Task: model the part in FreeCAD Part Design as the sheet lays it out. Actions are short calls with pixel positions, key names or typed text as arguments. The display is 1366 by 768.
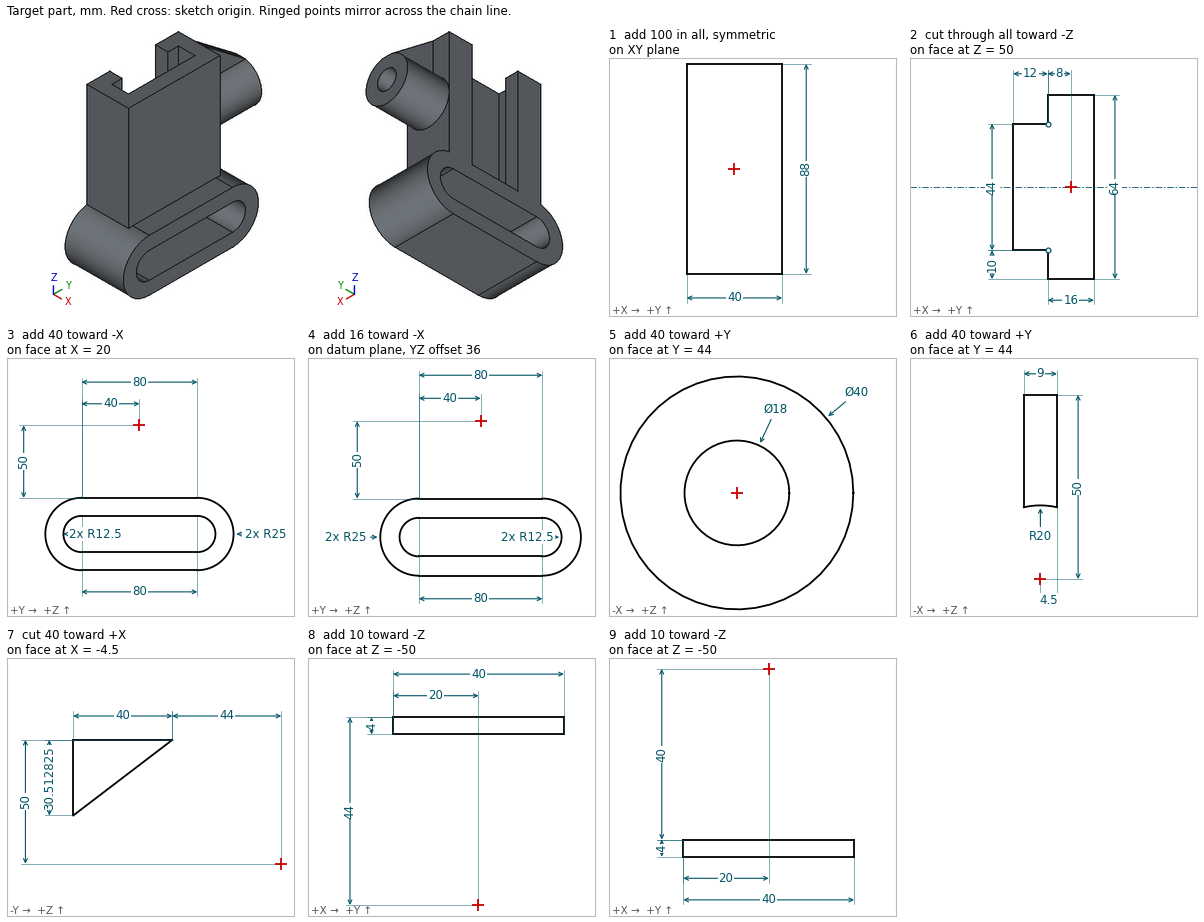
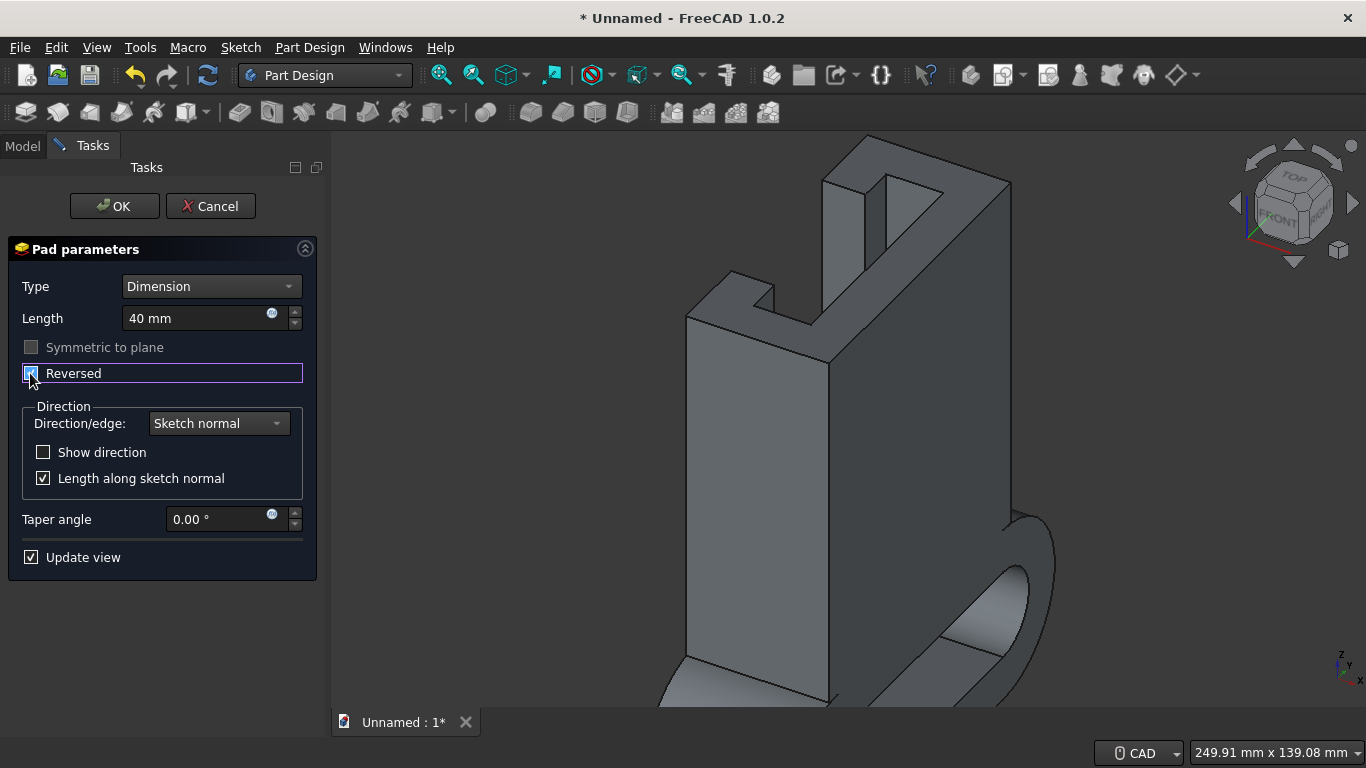
click(115, 206)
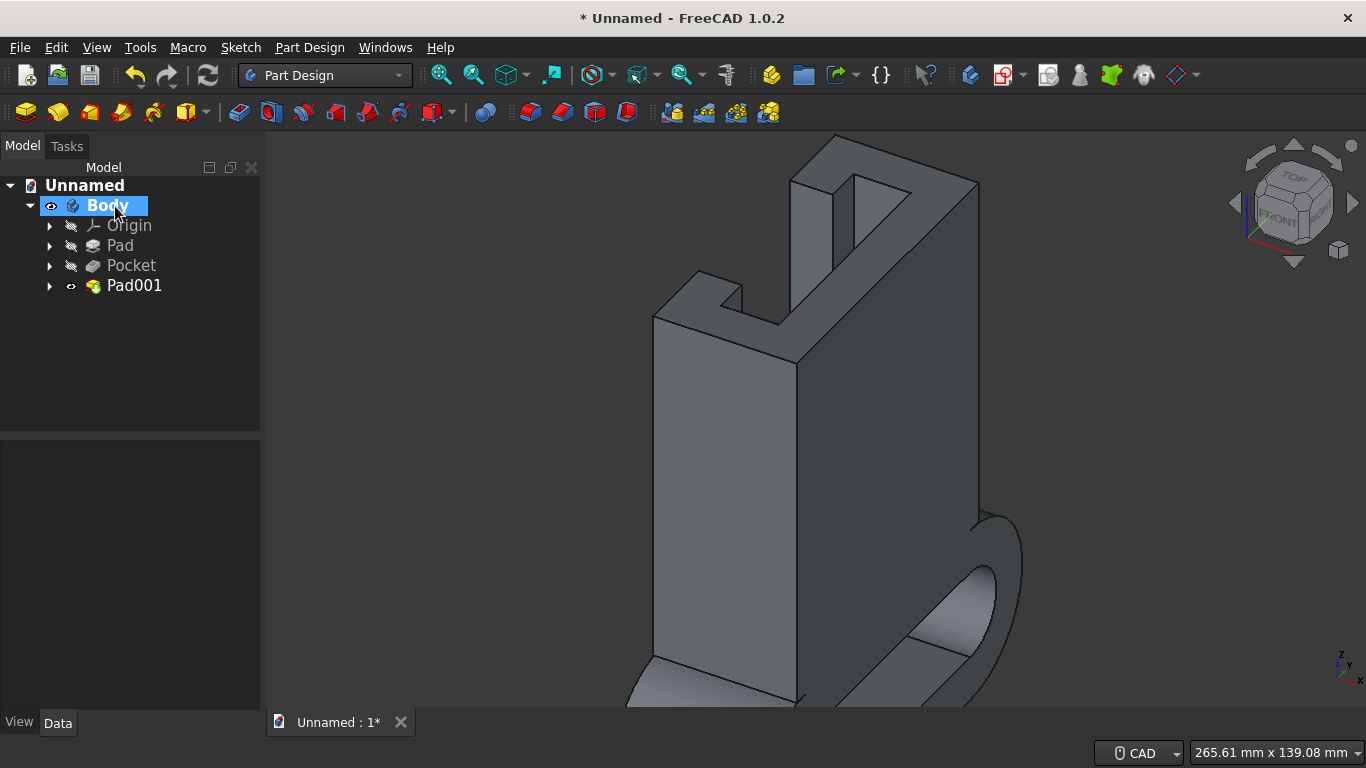
click(442, 76)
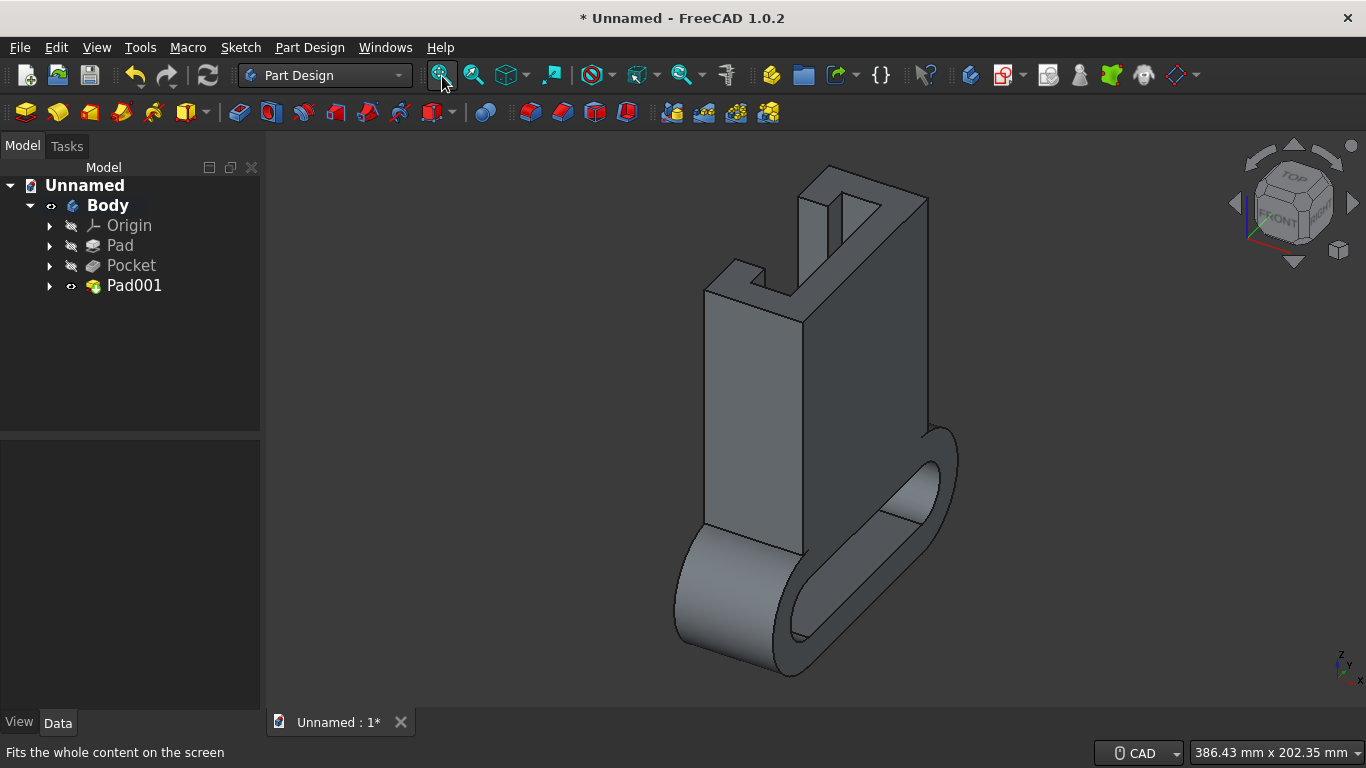
click(50, 226)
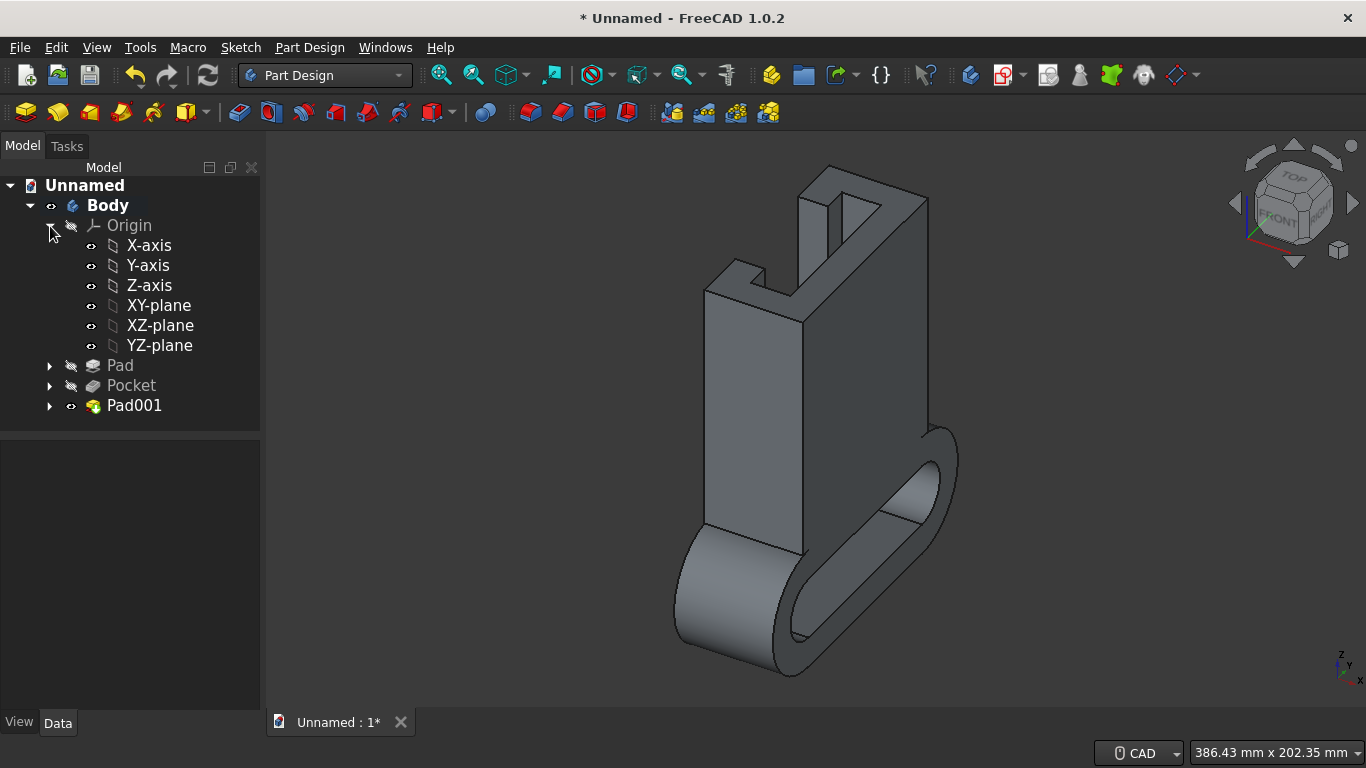
click(136, 346)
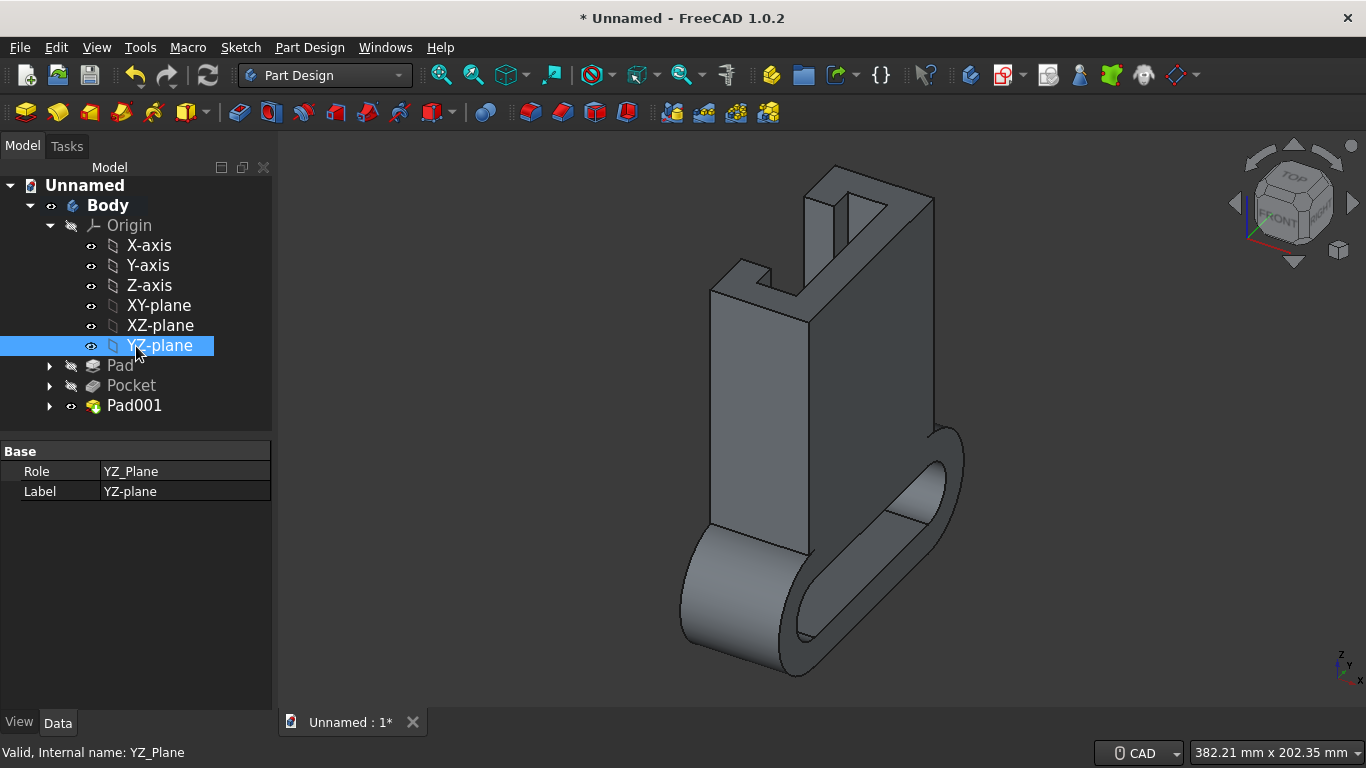
click(1176, 76)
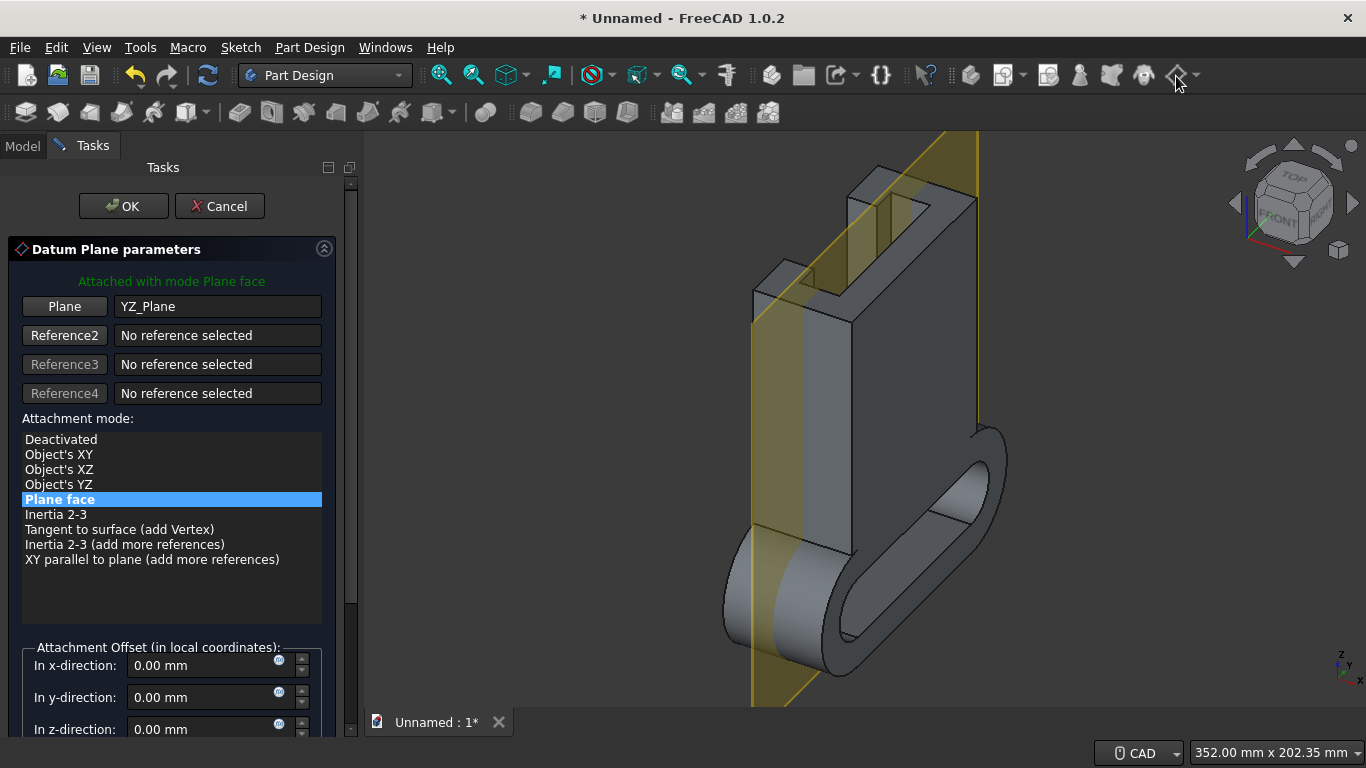
scroll(351, 456, down, 2)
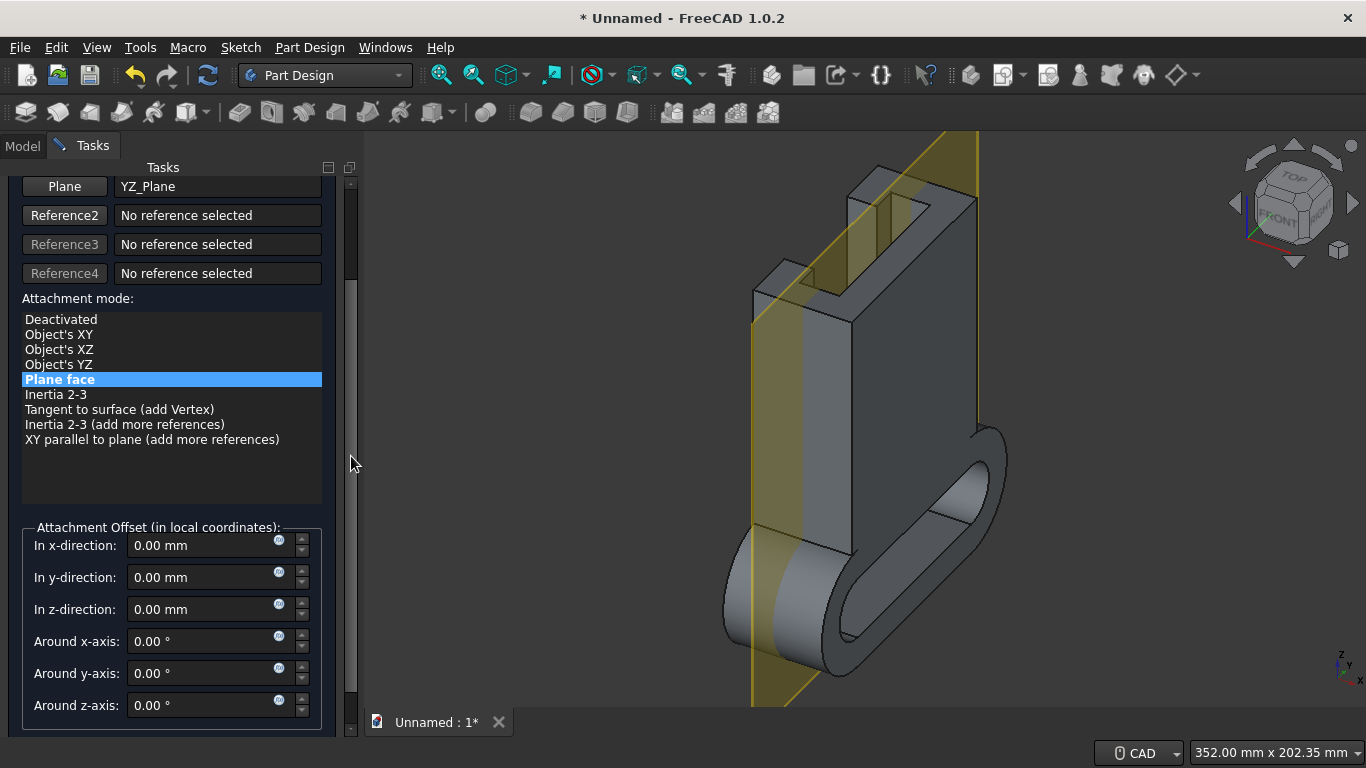
triple_click(210, 609)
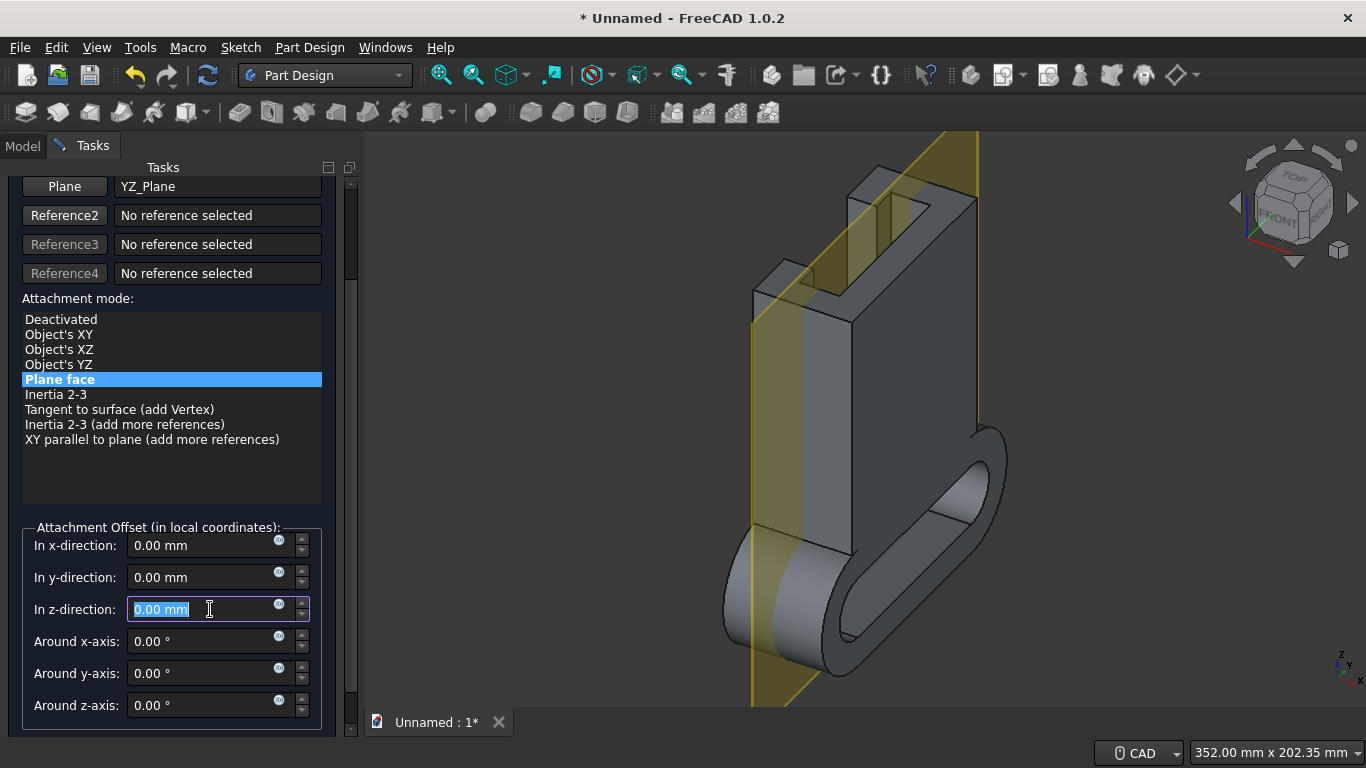
text(36)
key(Tab)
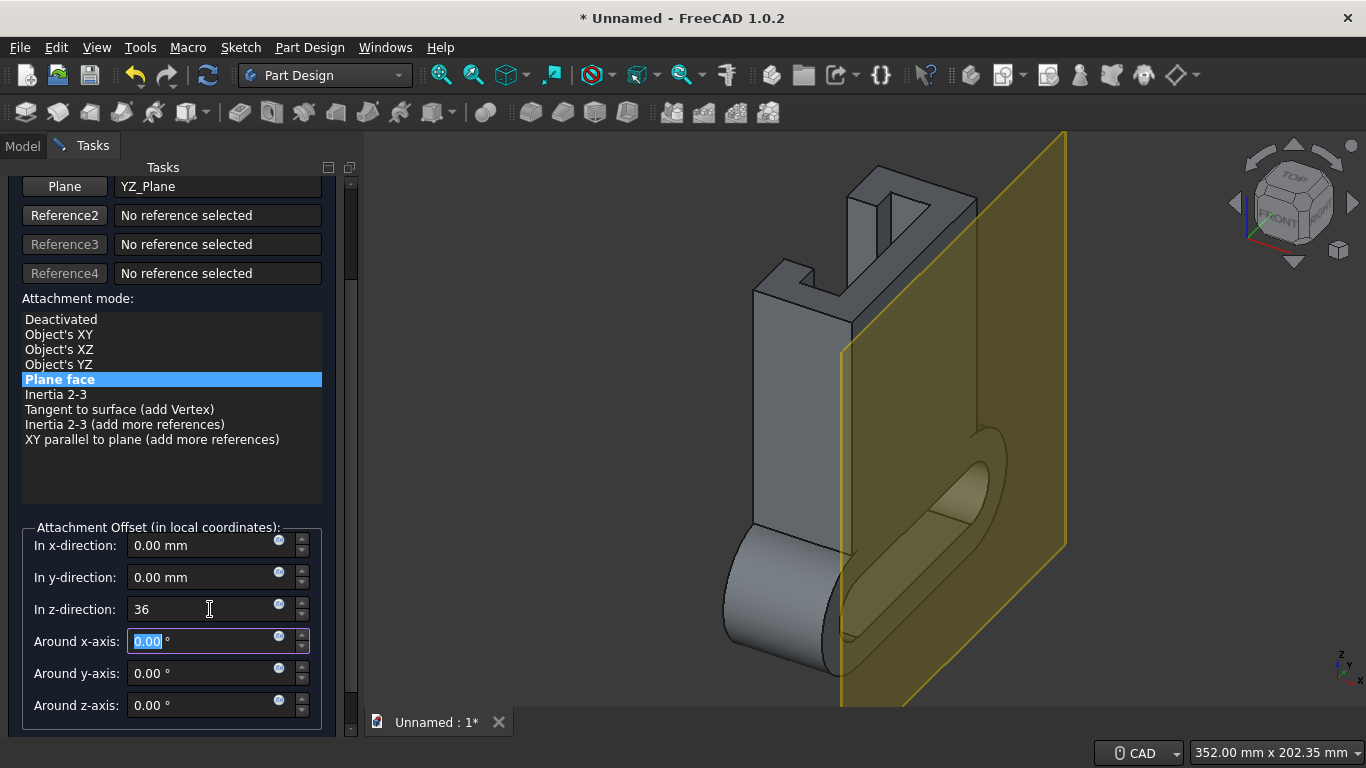
scroll(351, 456, up, 3)